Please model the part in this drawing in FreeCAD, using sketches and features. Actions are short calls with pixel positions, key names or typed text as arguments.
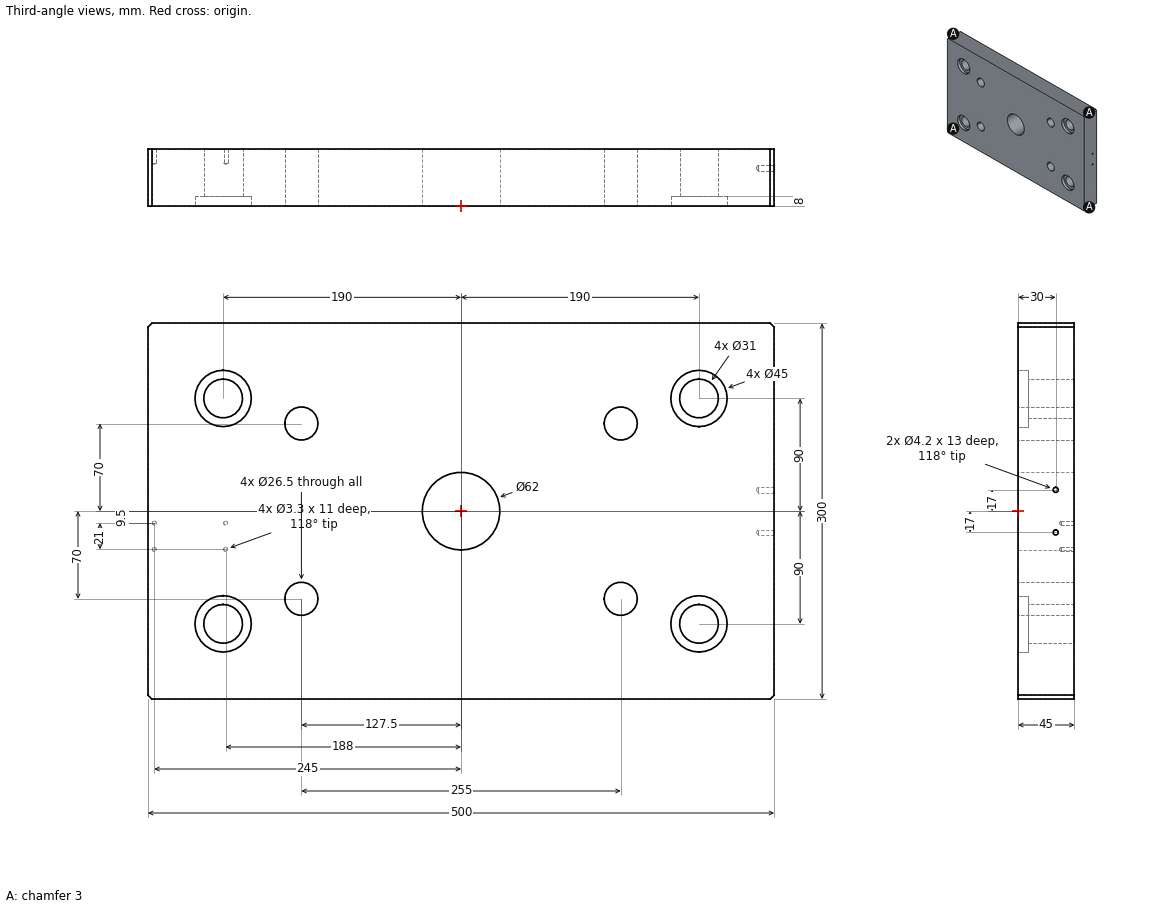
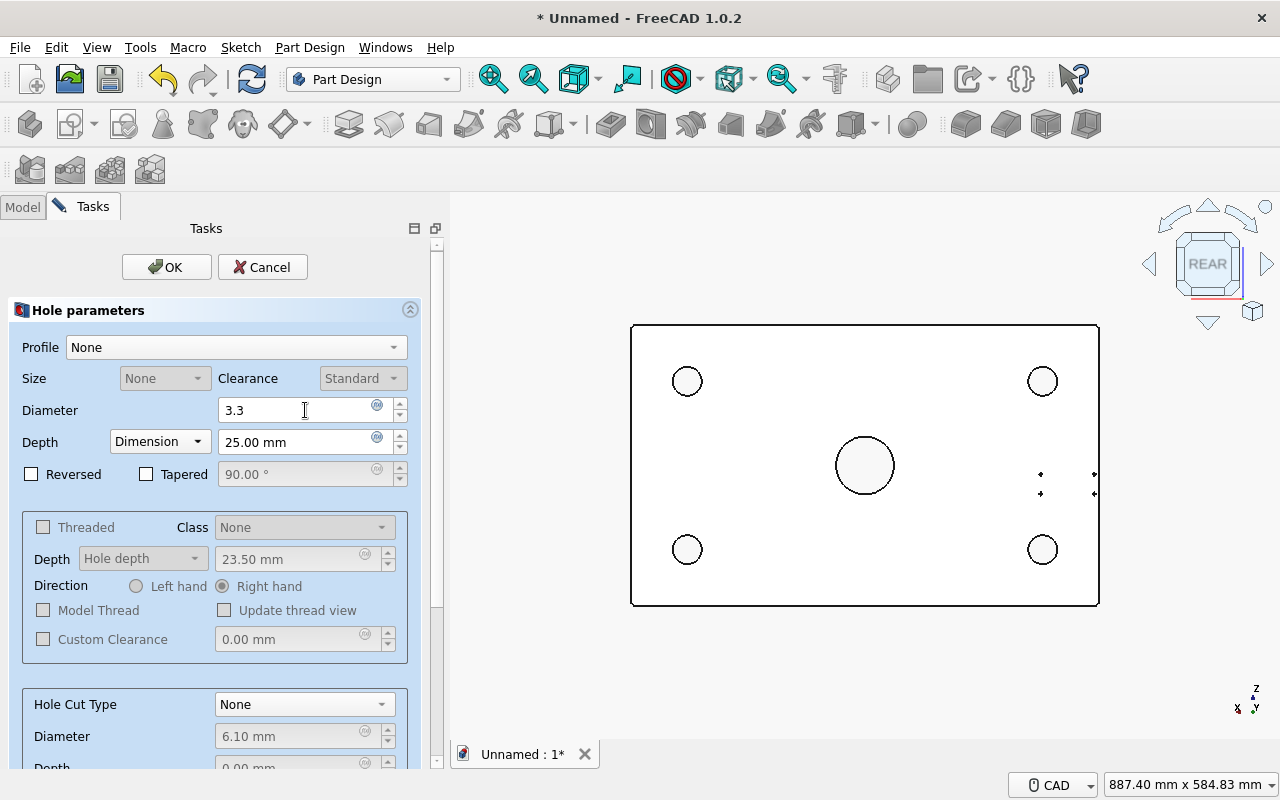
triple_click(305, 442)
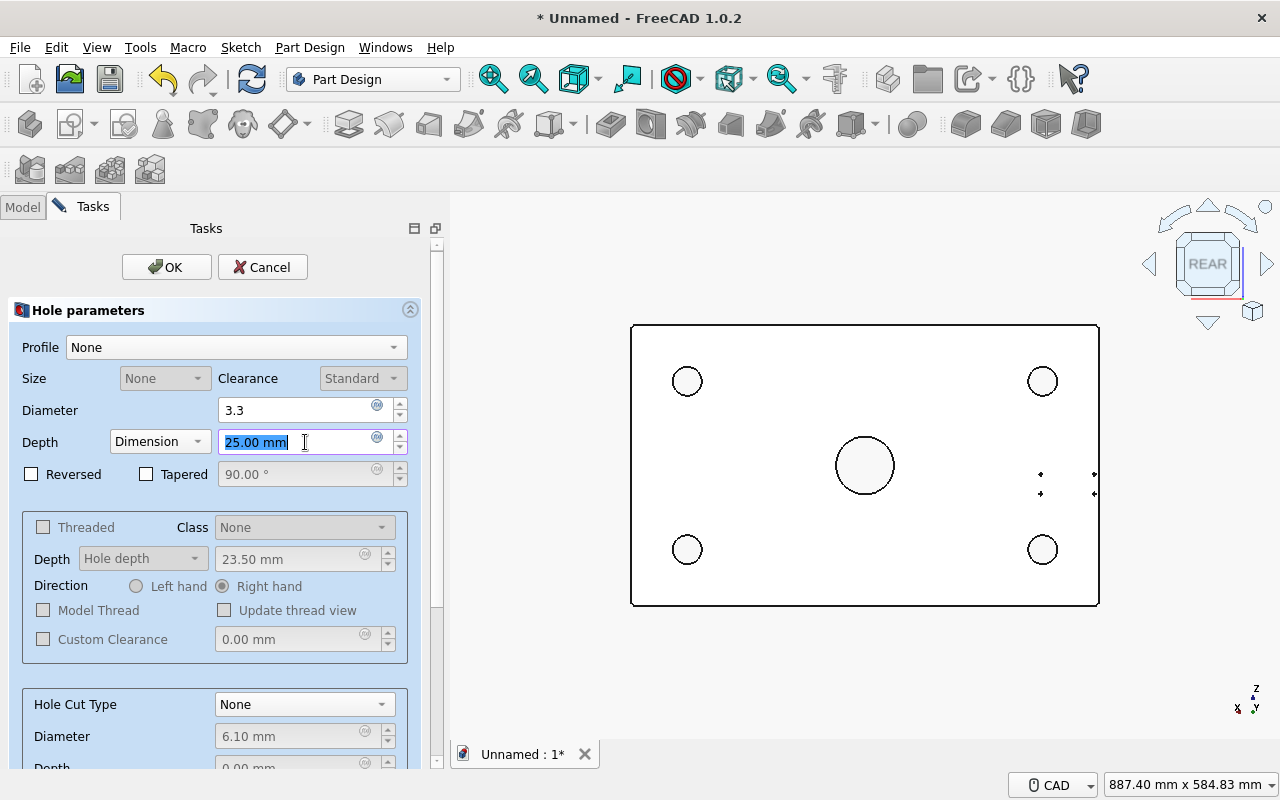
text(11)
key(Tab)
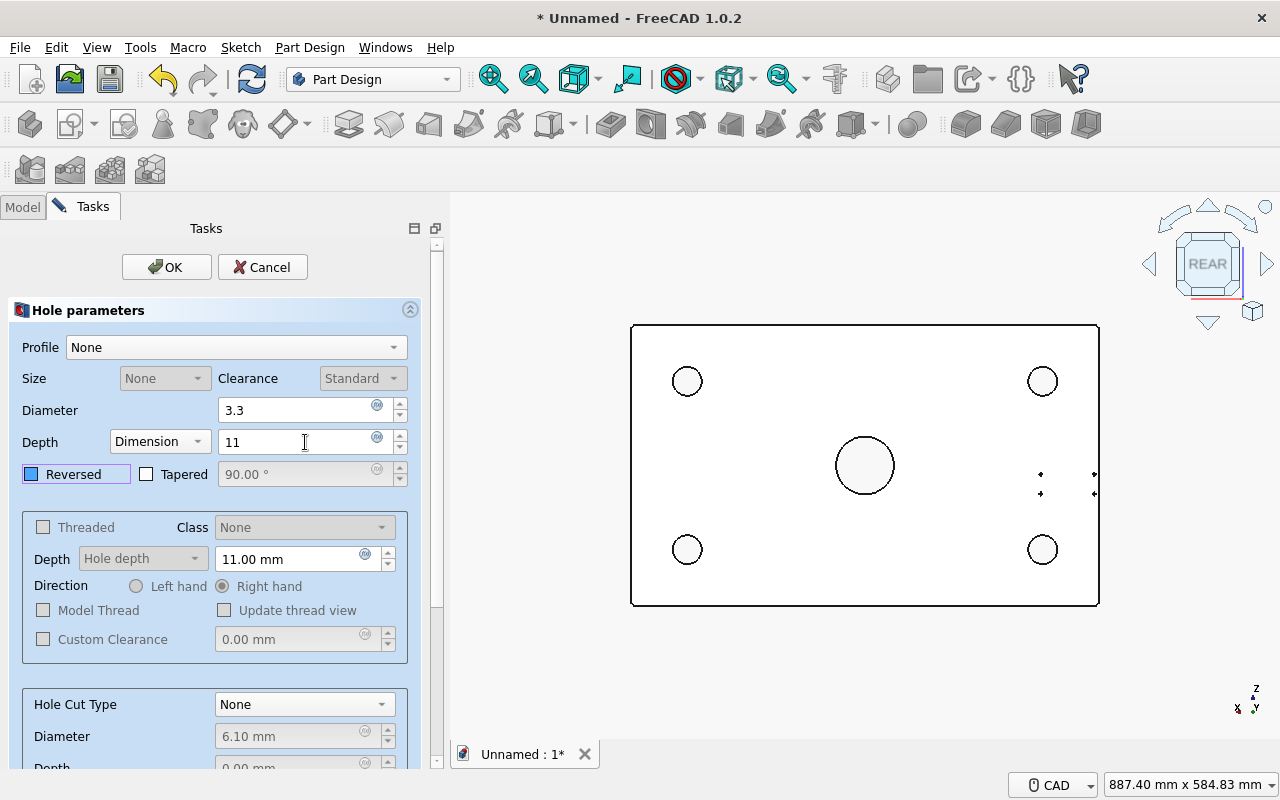
click(167, 267)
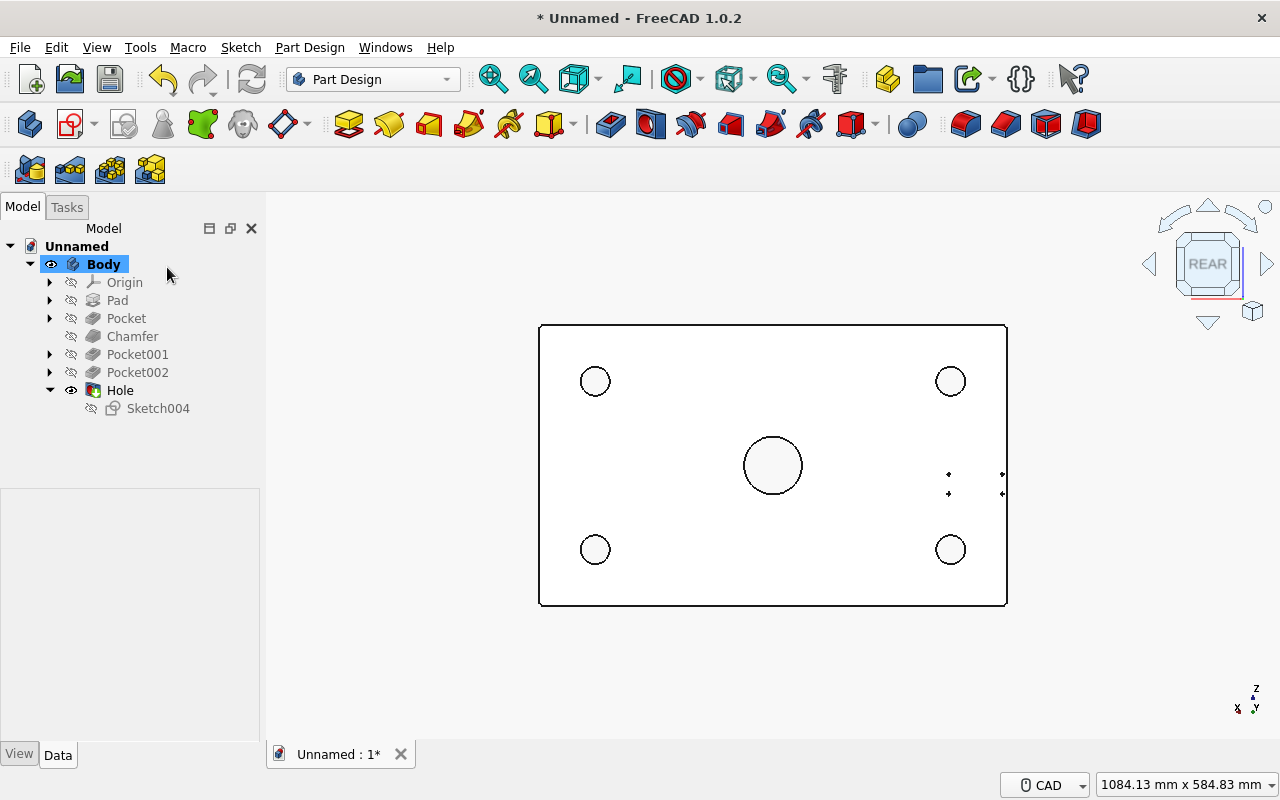
key(0)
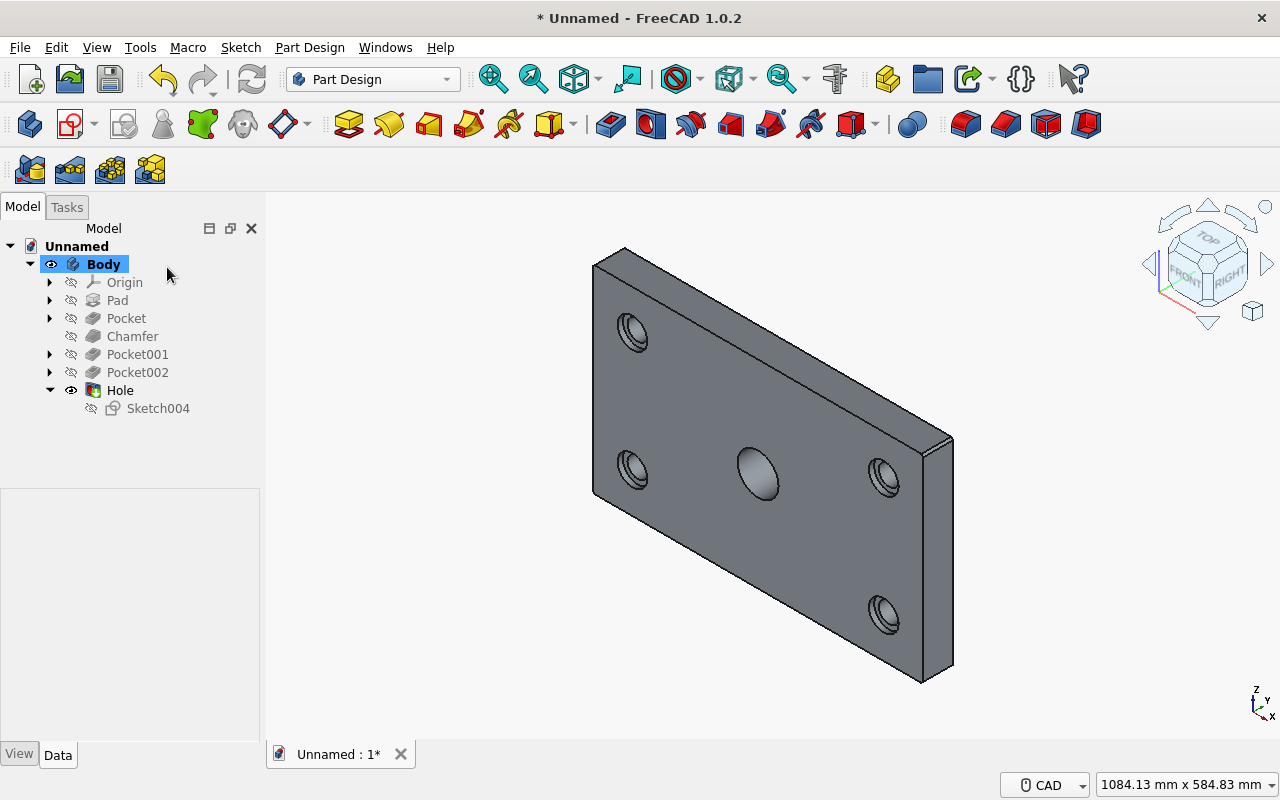
click(938, 560)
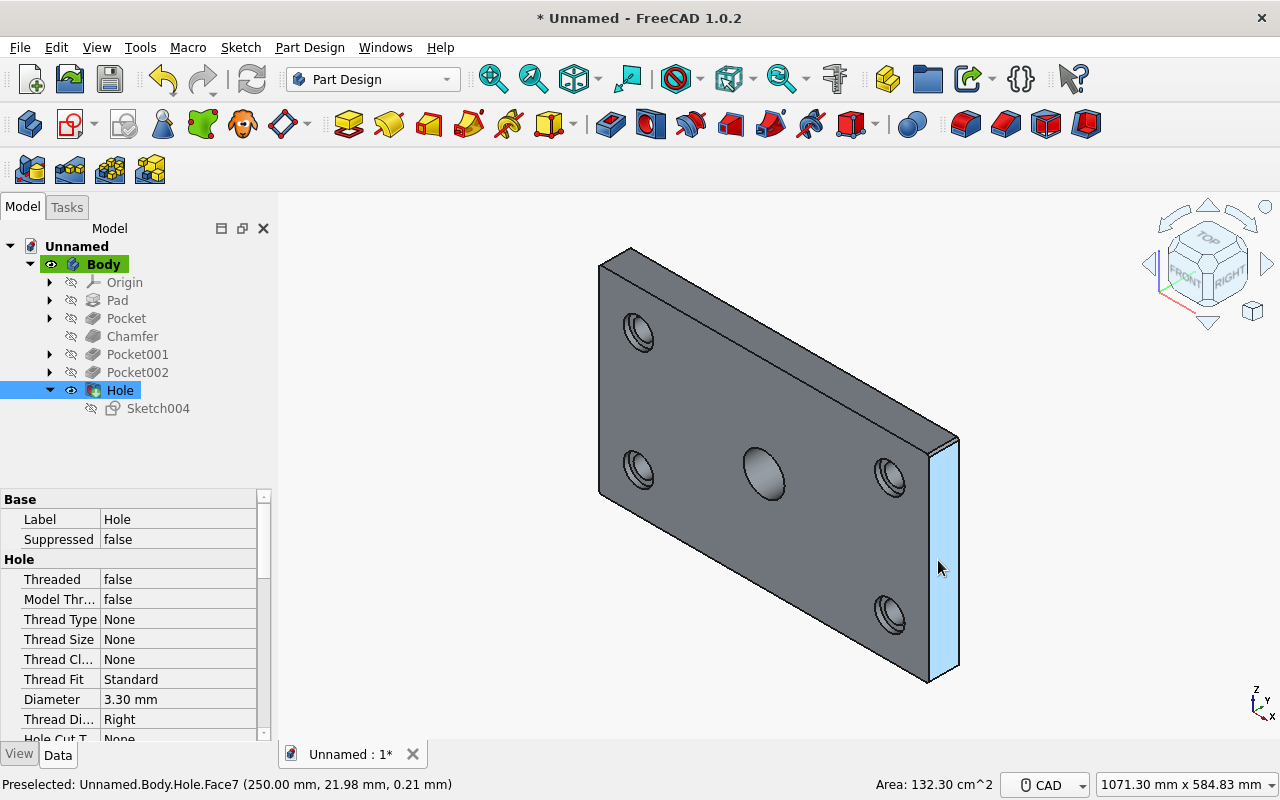
click(70, 124)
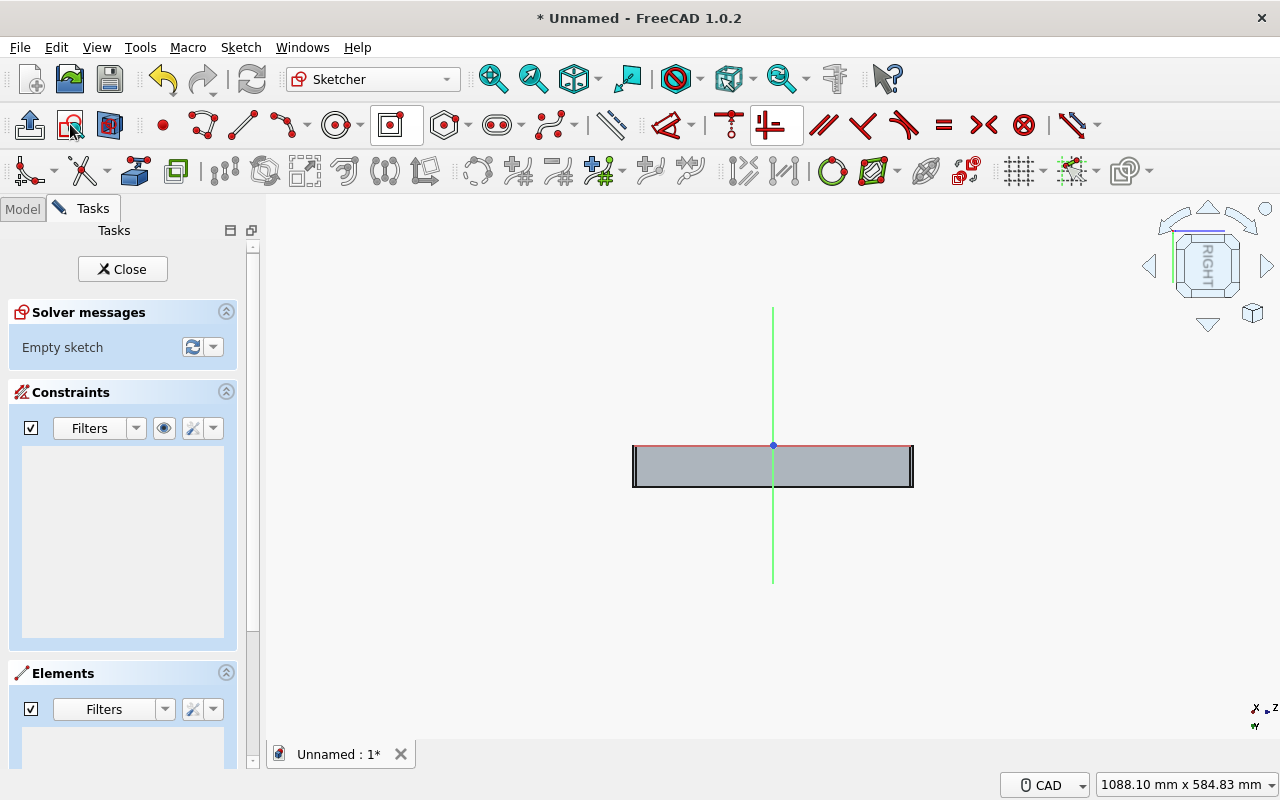
scroll(780, 460, up, 12)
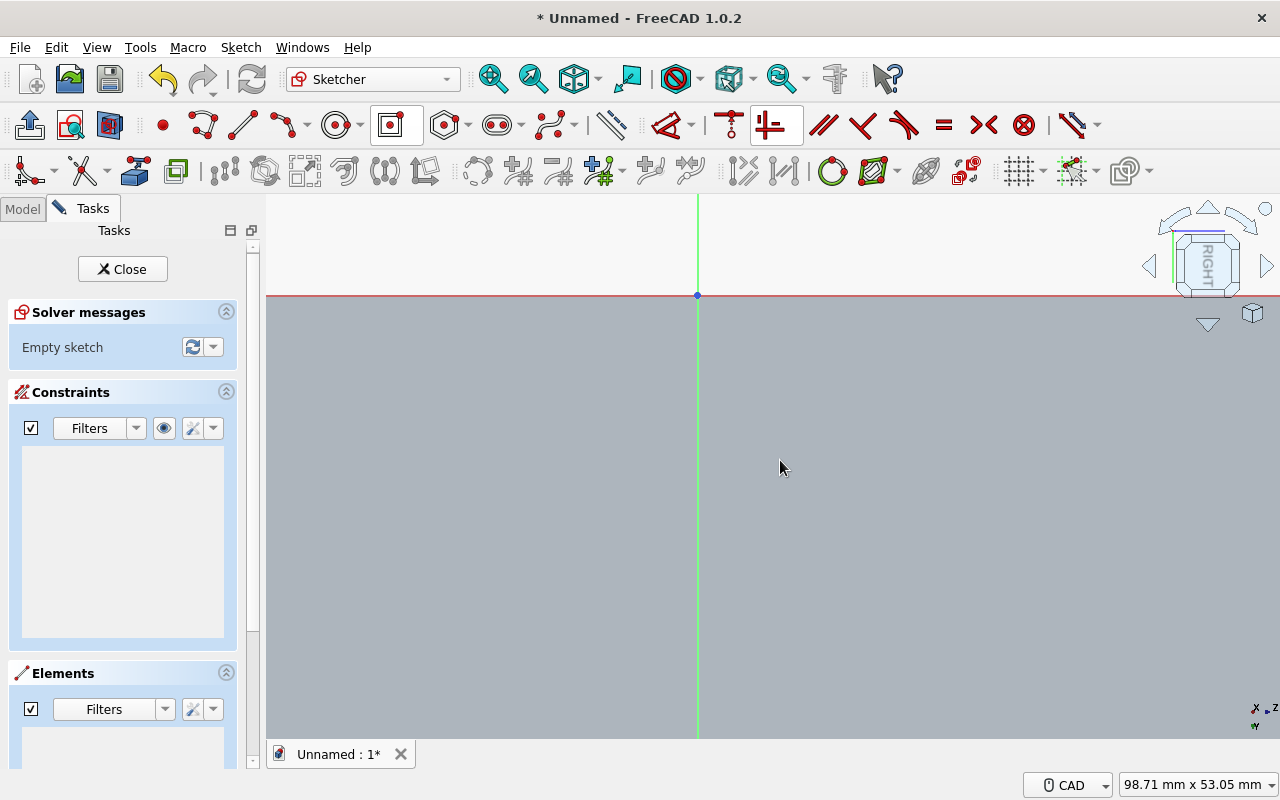
click(336, 126)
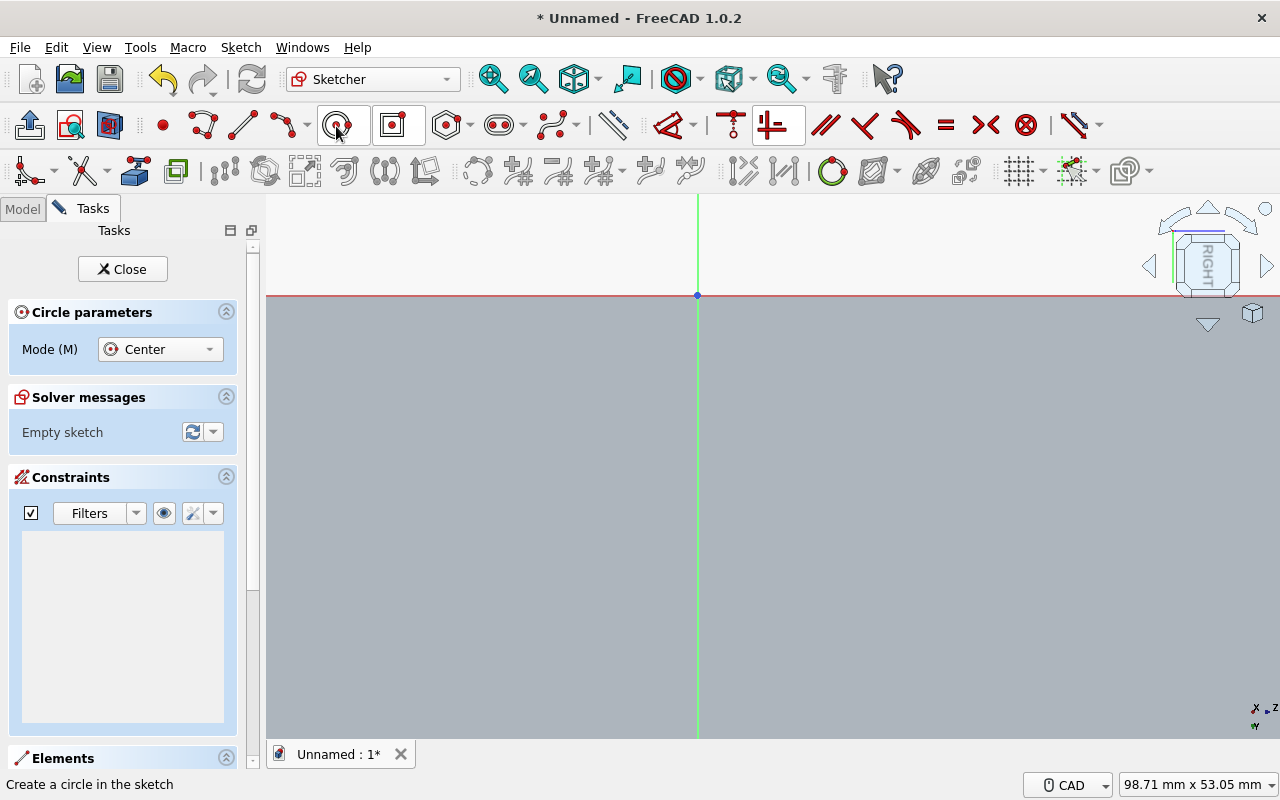
click(872, 604)
click(888, 589)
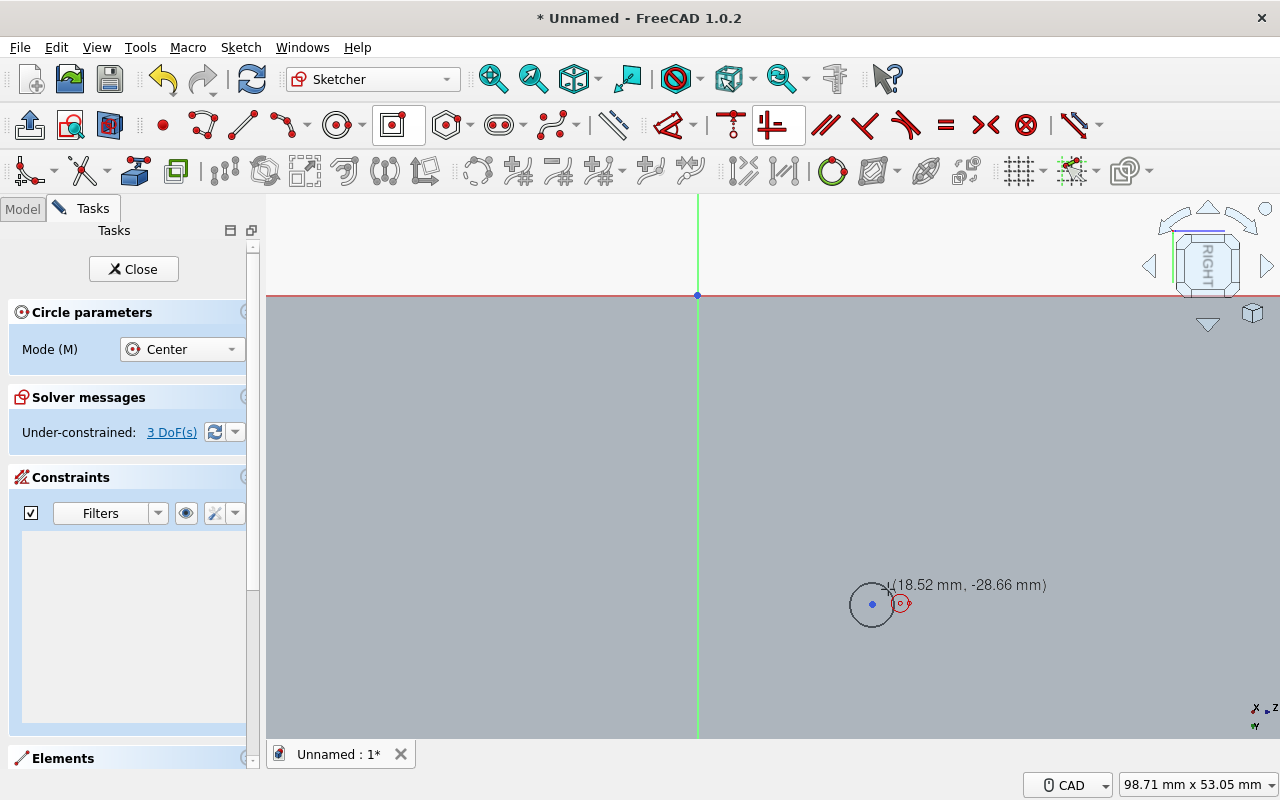
click(523, 604)
click(538, 589)
key(Escape)